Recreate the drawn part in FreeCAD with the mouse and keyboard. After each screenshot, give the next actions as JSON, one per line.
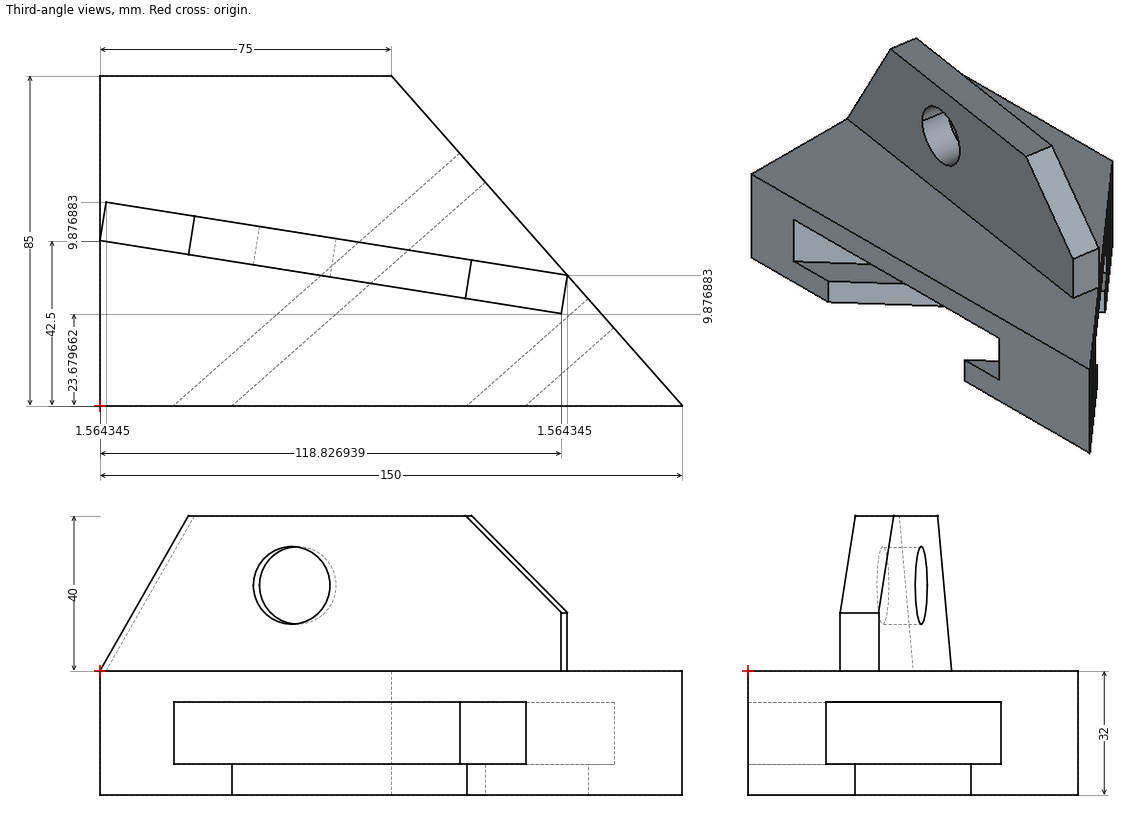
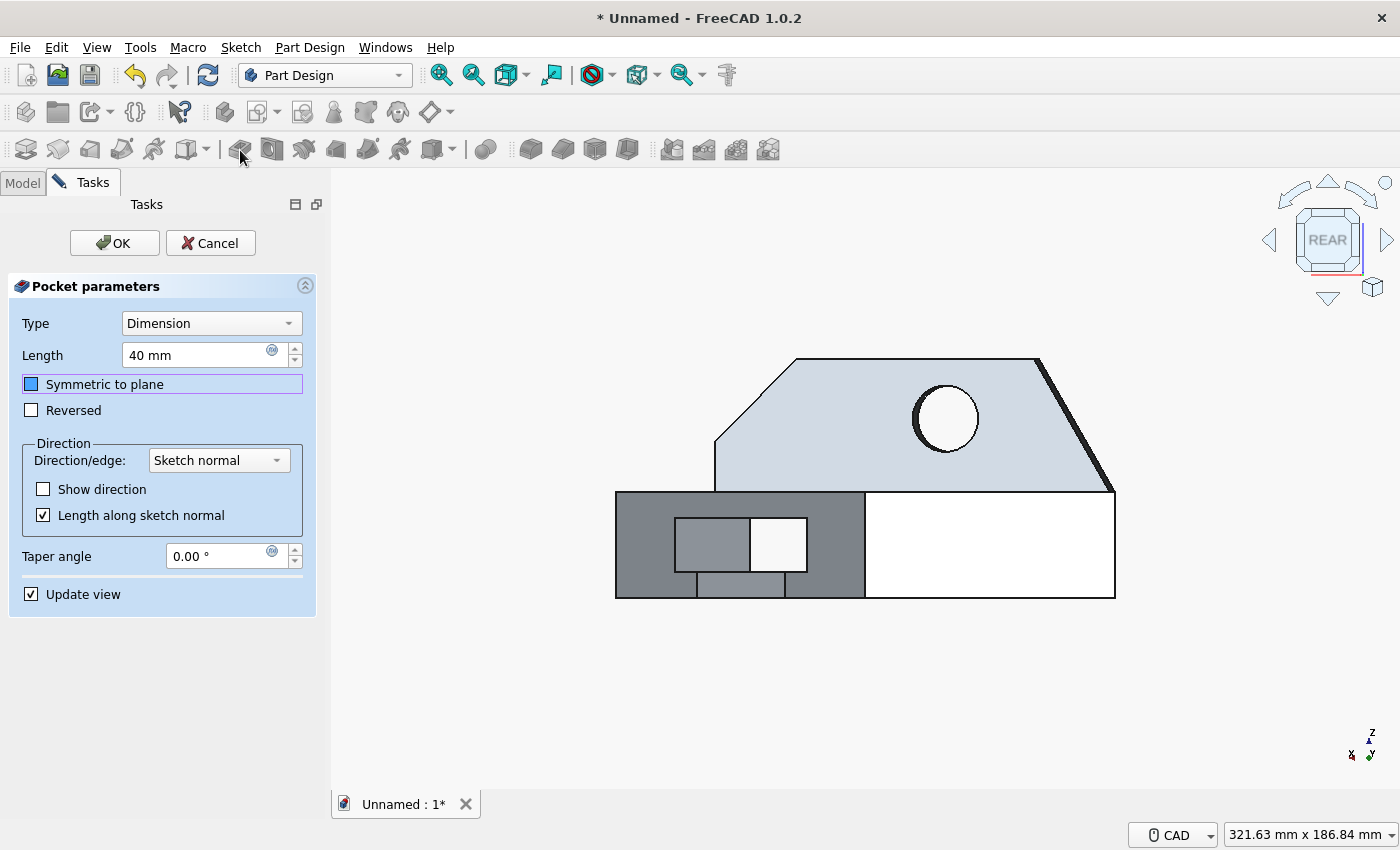
{"action": "left_click", "coordinate": [115, 243]}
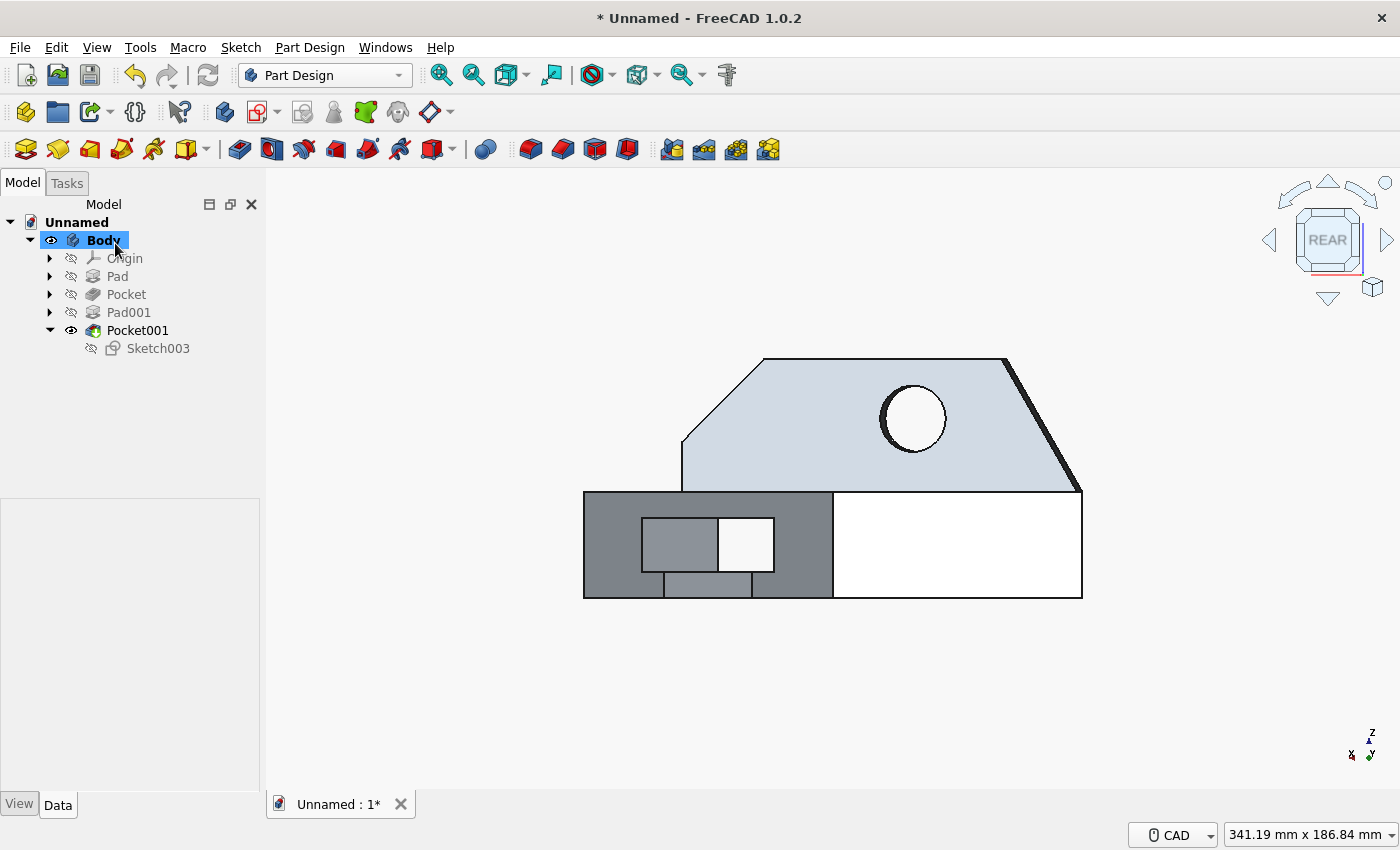
{"action": "key", "text": "0"}